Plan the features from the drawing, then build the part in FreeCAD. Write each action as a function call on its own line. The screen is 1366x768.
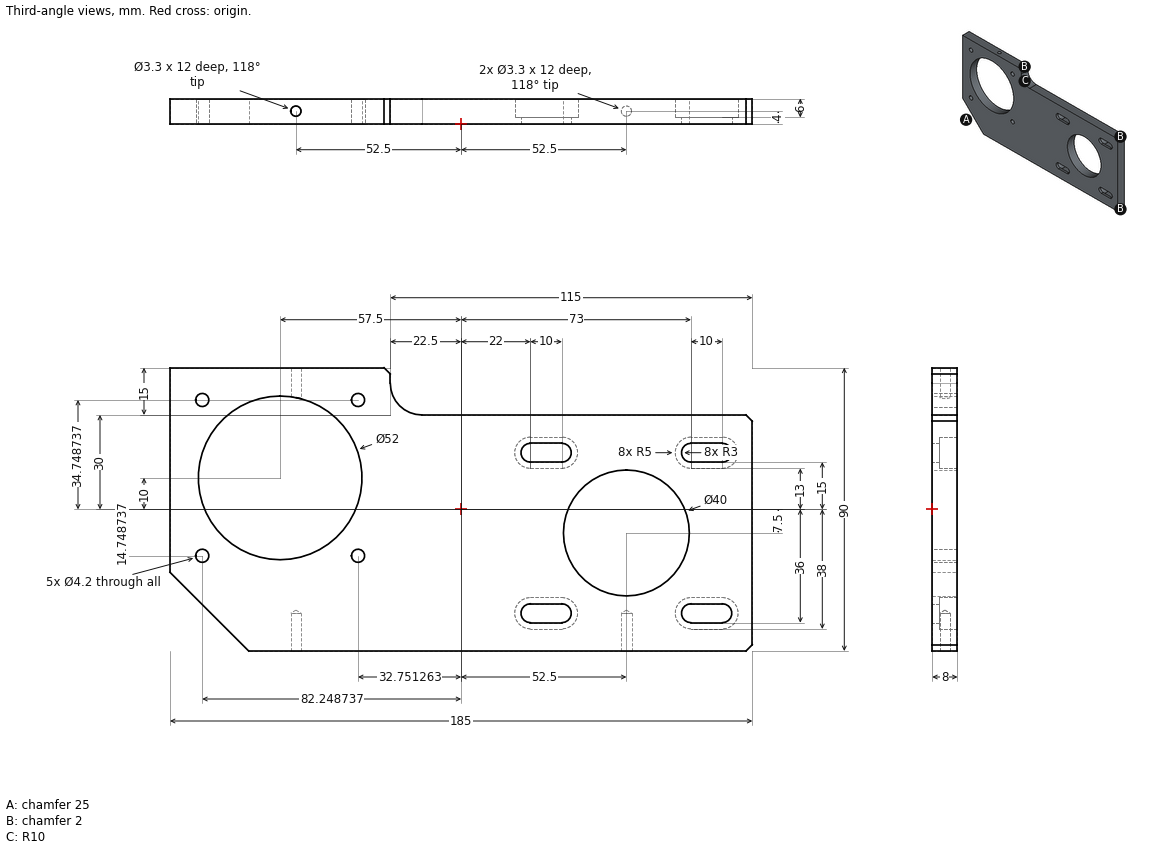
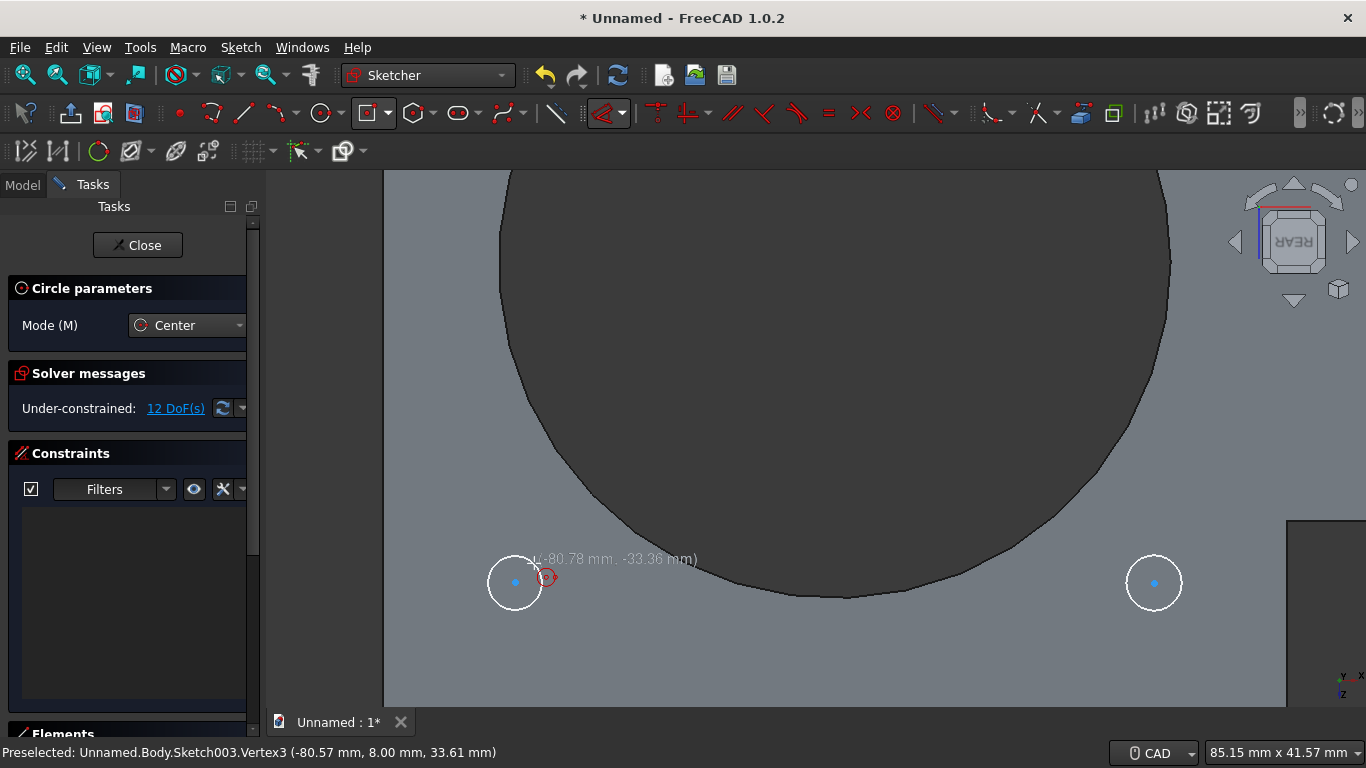
click(835, 262)
click(854, 243)
key(Escape)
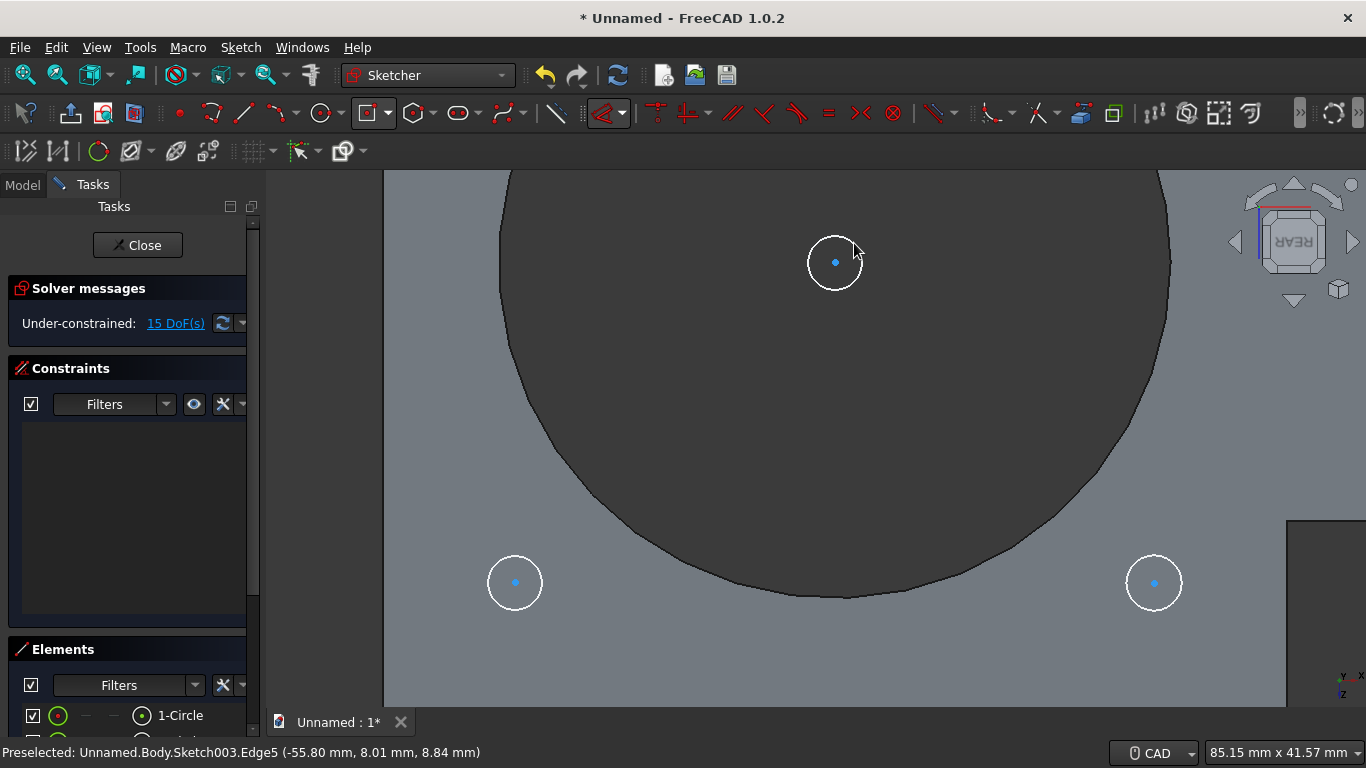
scroll(515, 582, down, 4)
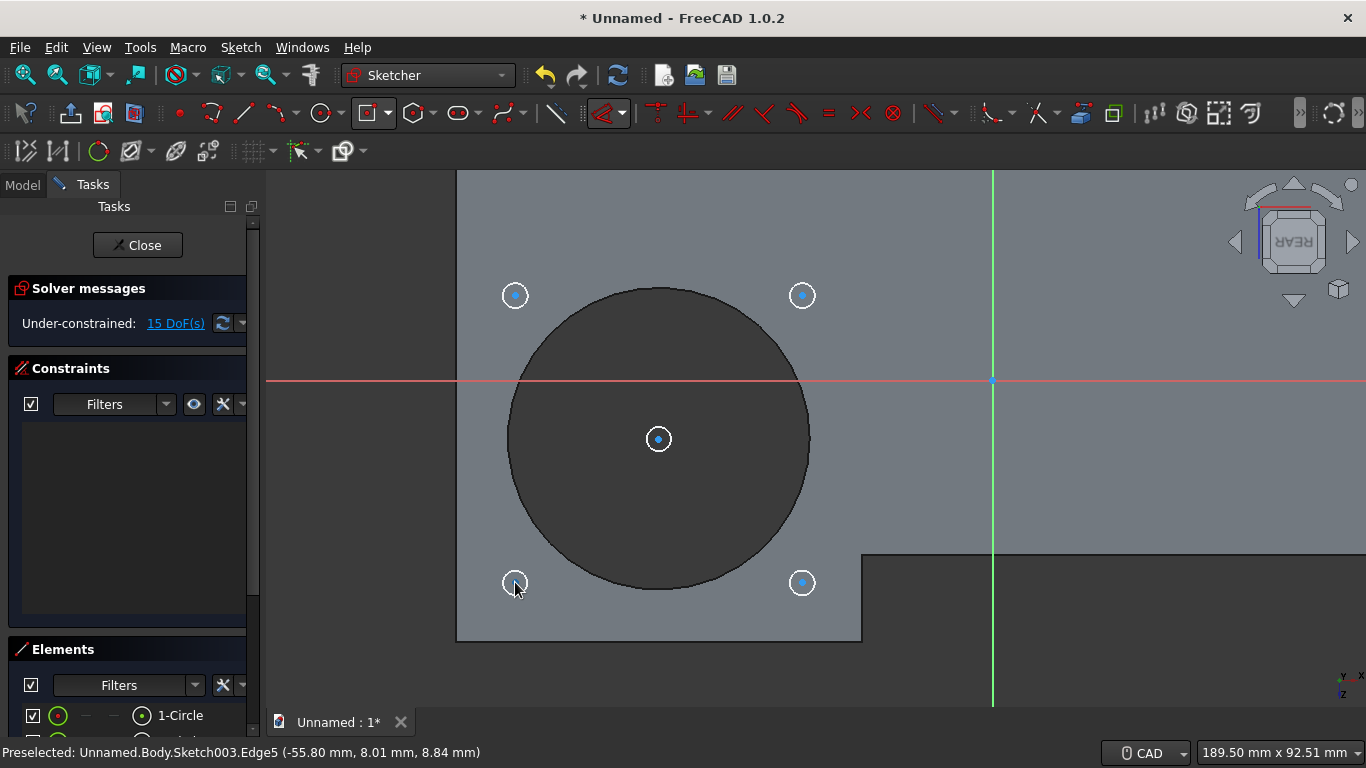
click(524, 287)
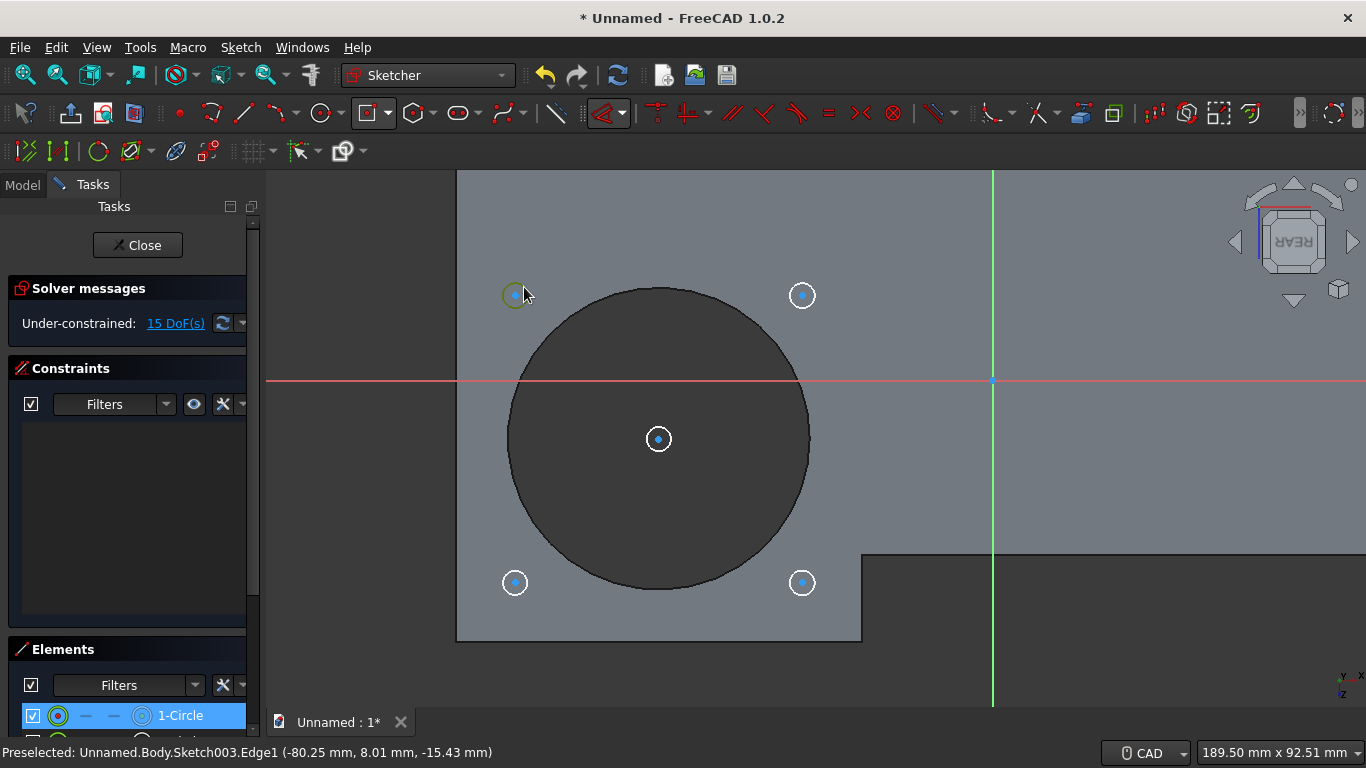
click(811, 287)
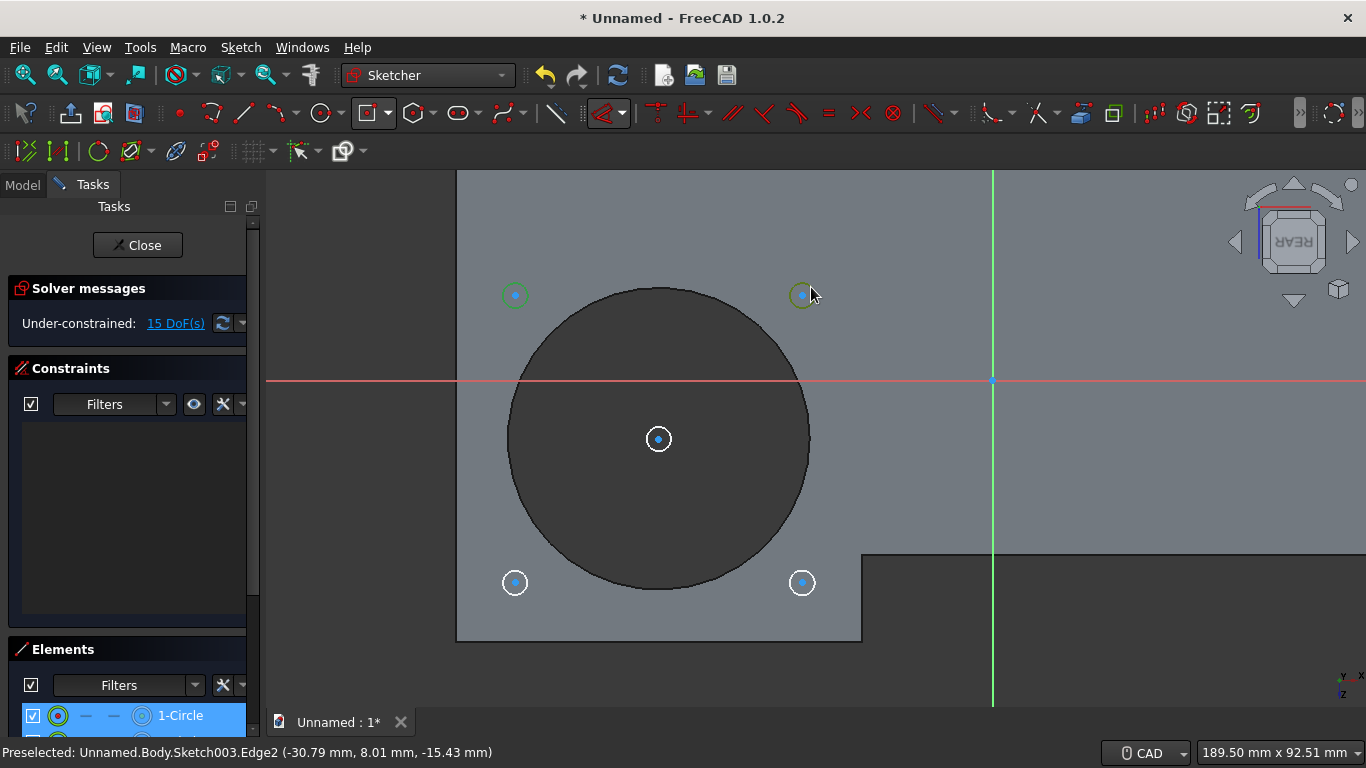
click(811, 574)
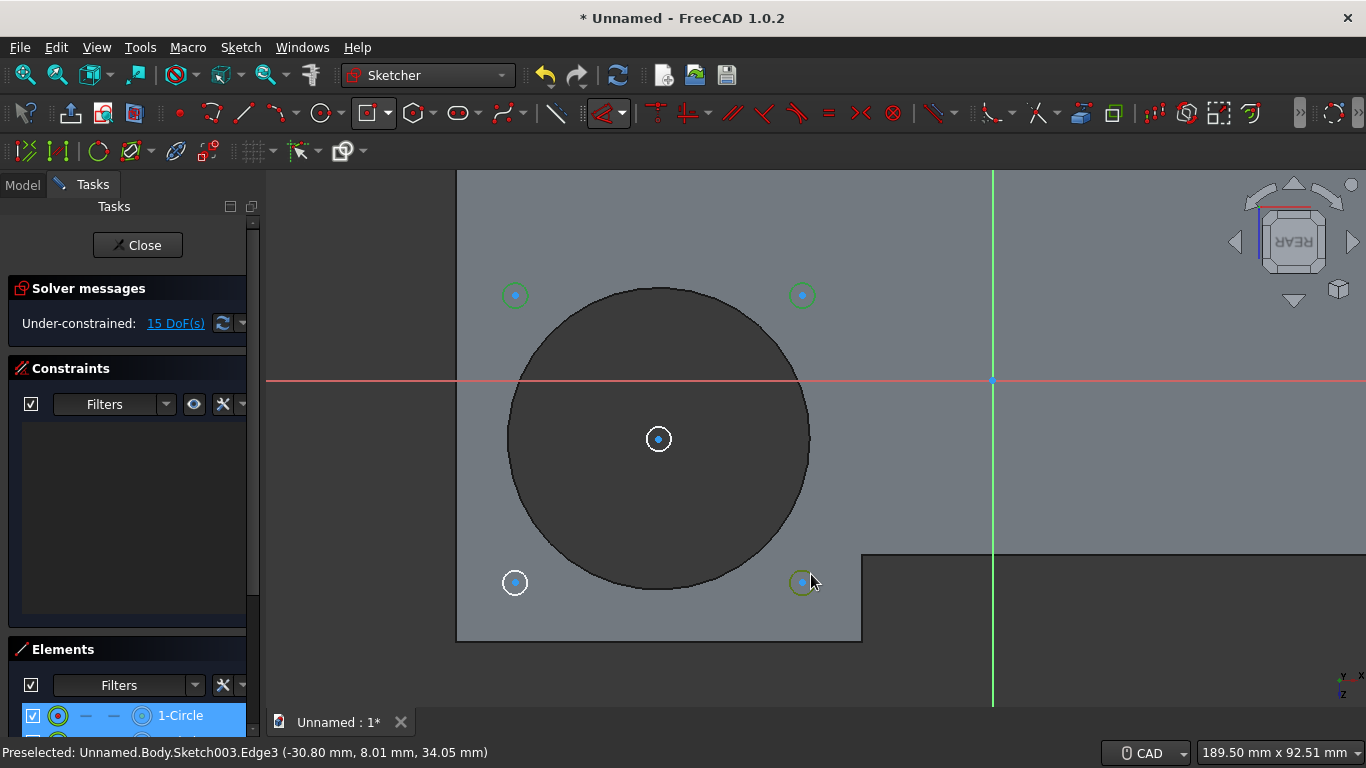
click(524, 574)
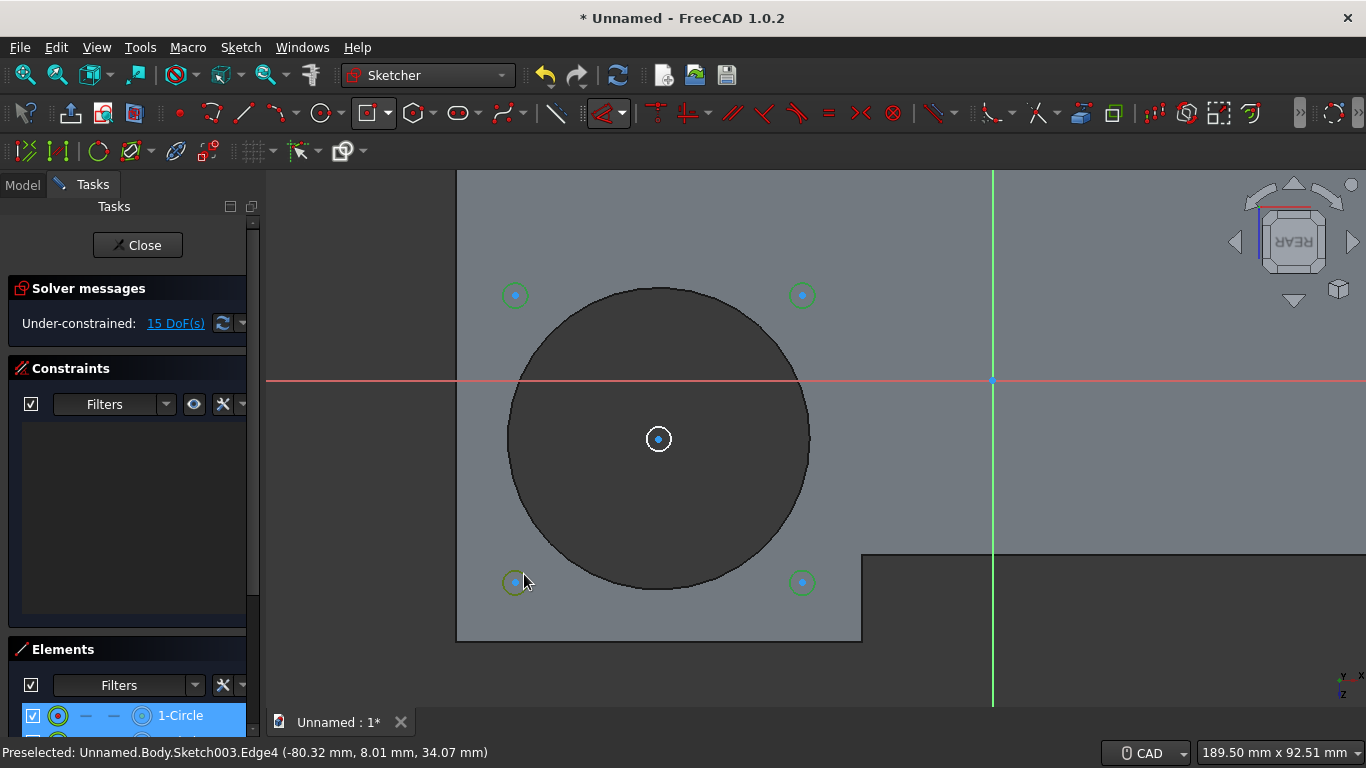
click(667, 431)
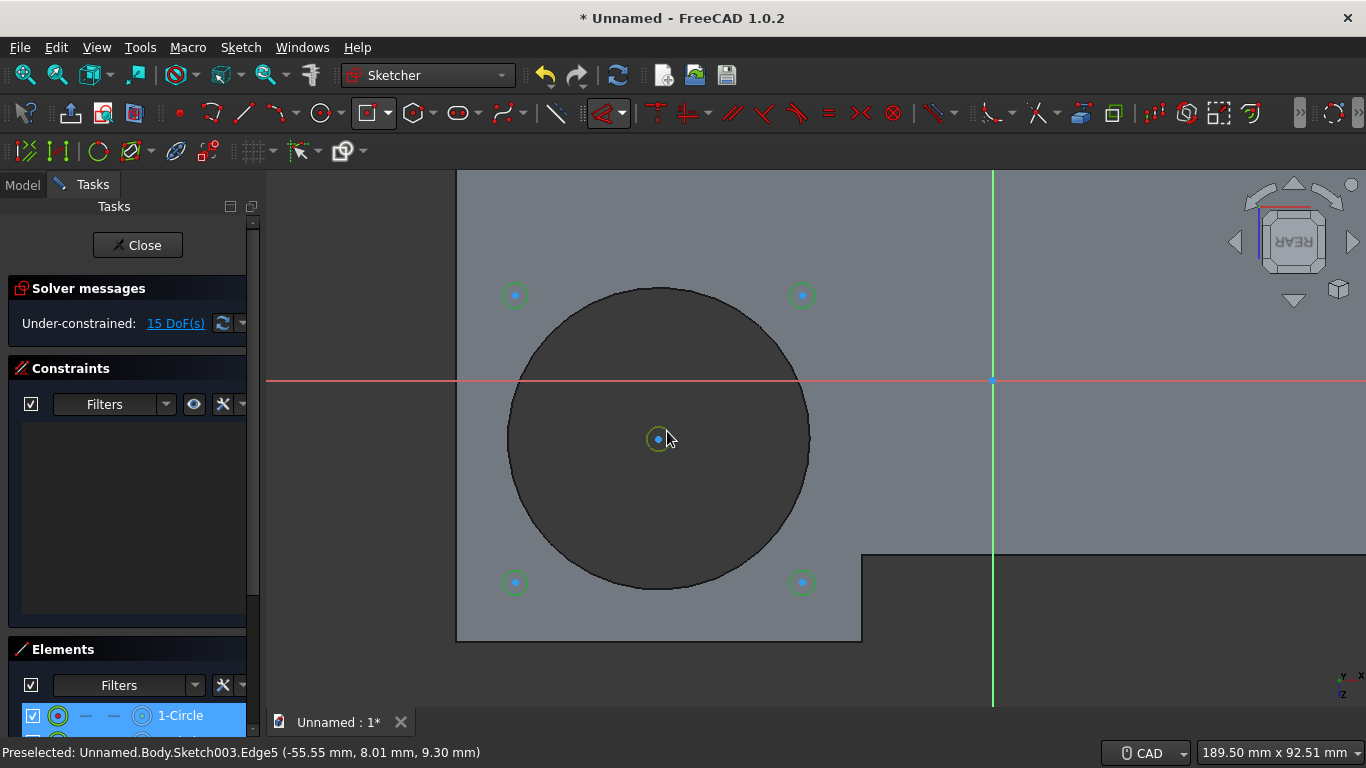
click(830, 114)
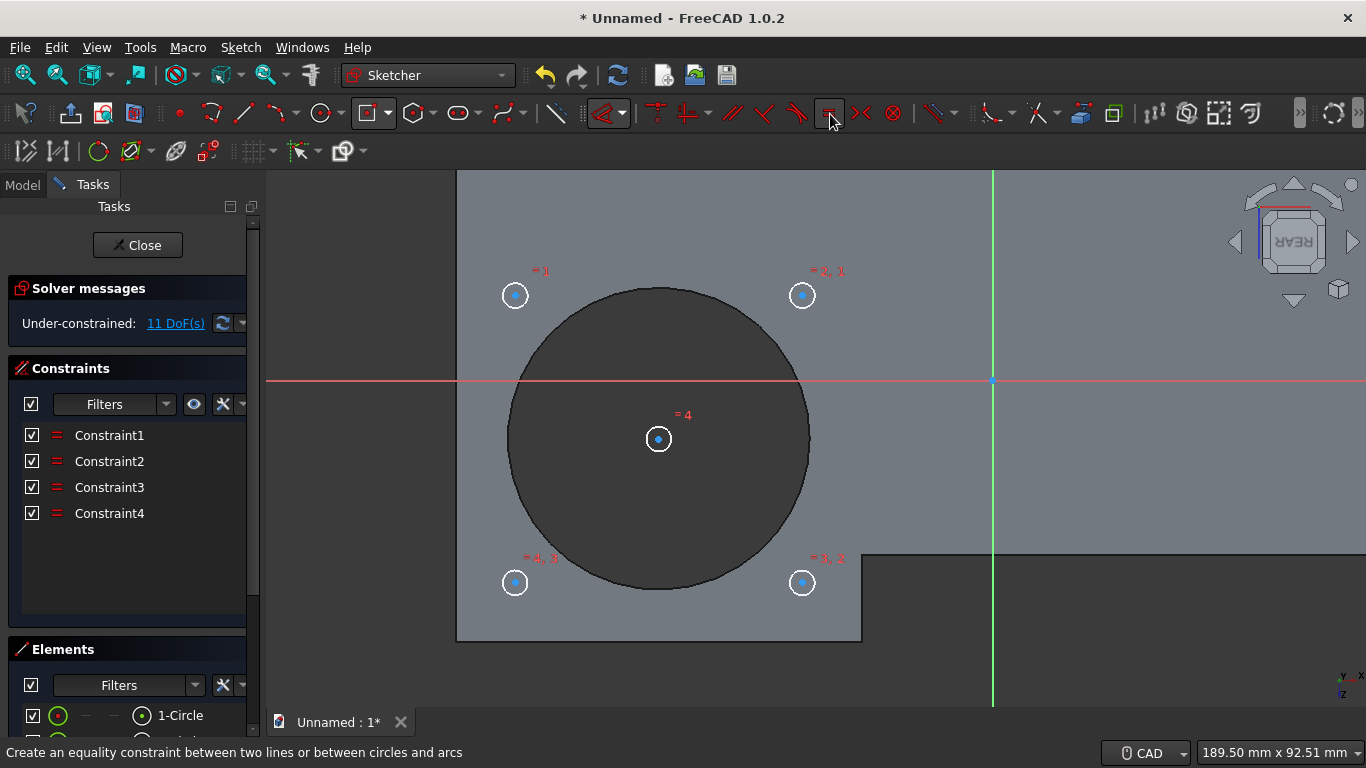
click(515, 296)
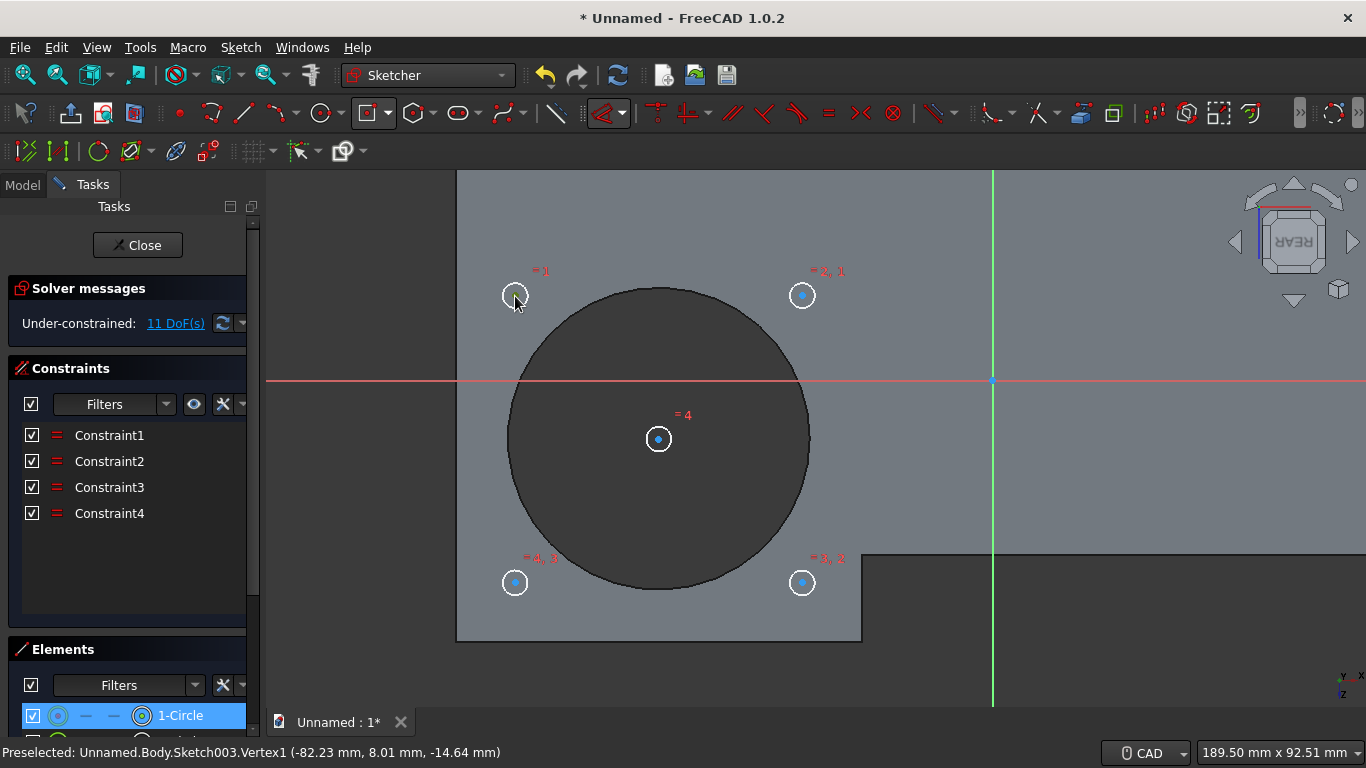
click(802, 296)